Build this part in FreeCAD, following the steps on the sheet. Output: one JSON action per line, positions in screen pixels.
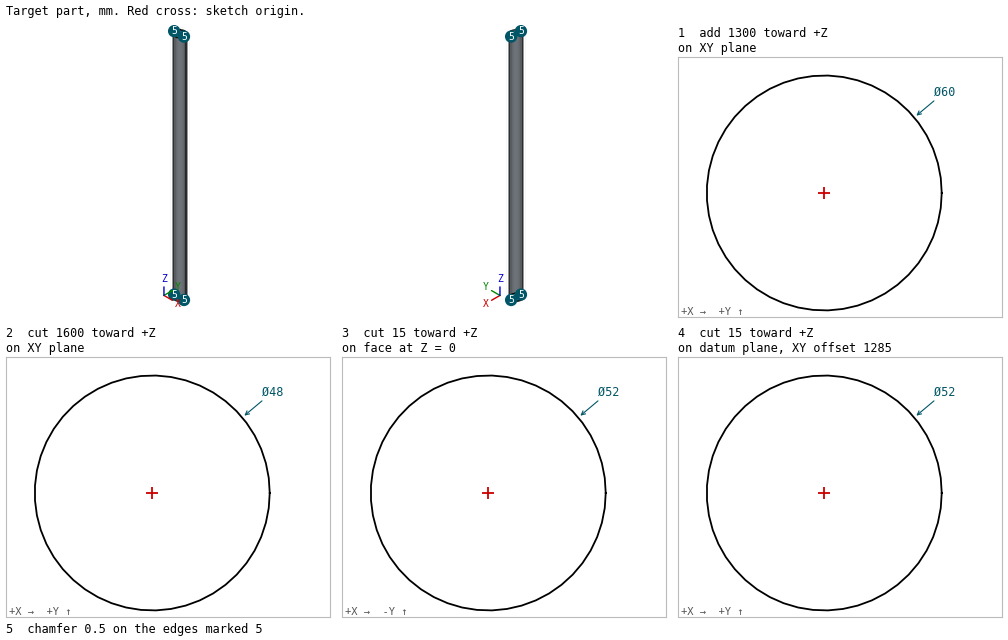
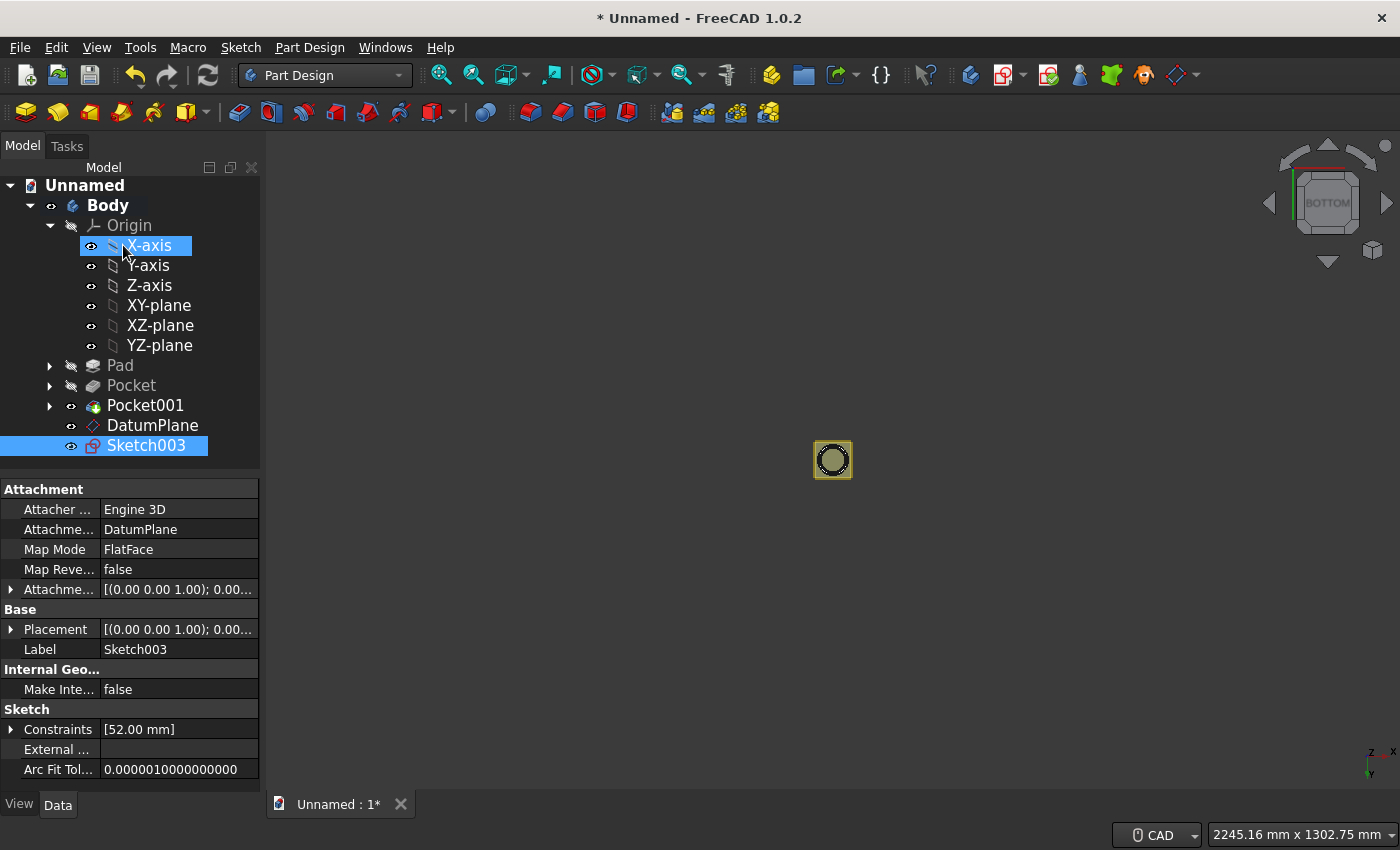
{"action": "left_click", "coordinate": [240, 112]}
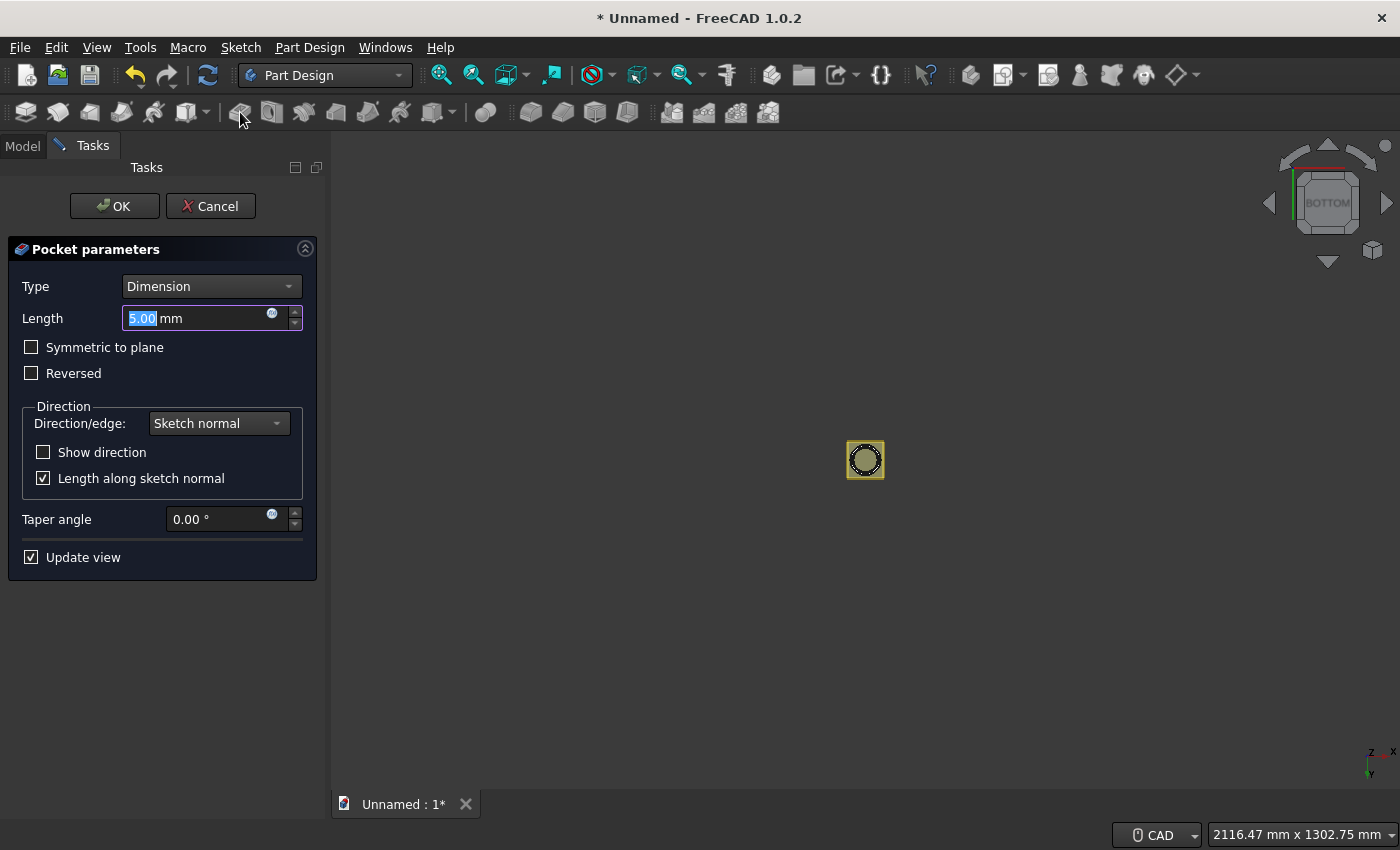
{"action": "type", "text": "15"}
{"action": "key", "text": "Tab"}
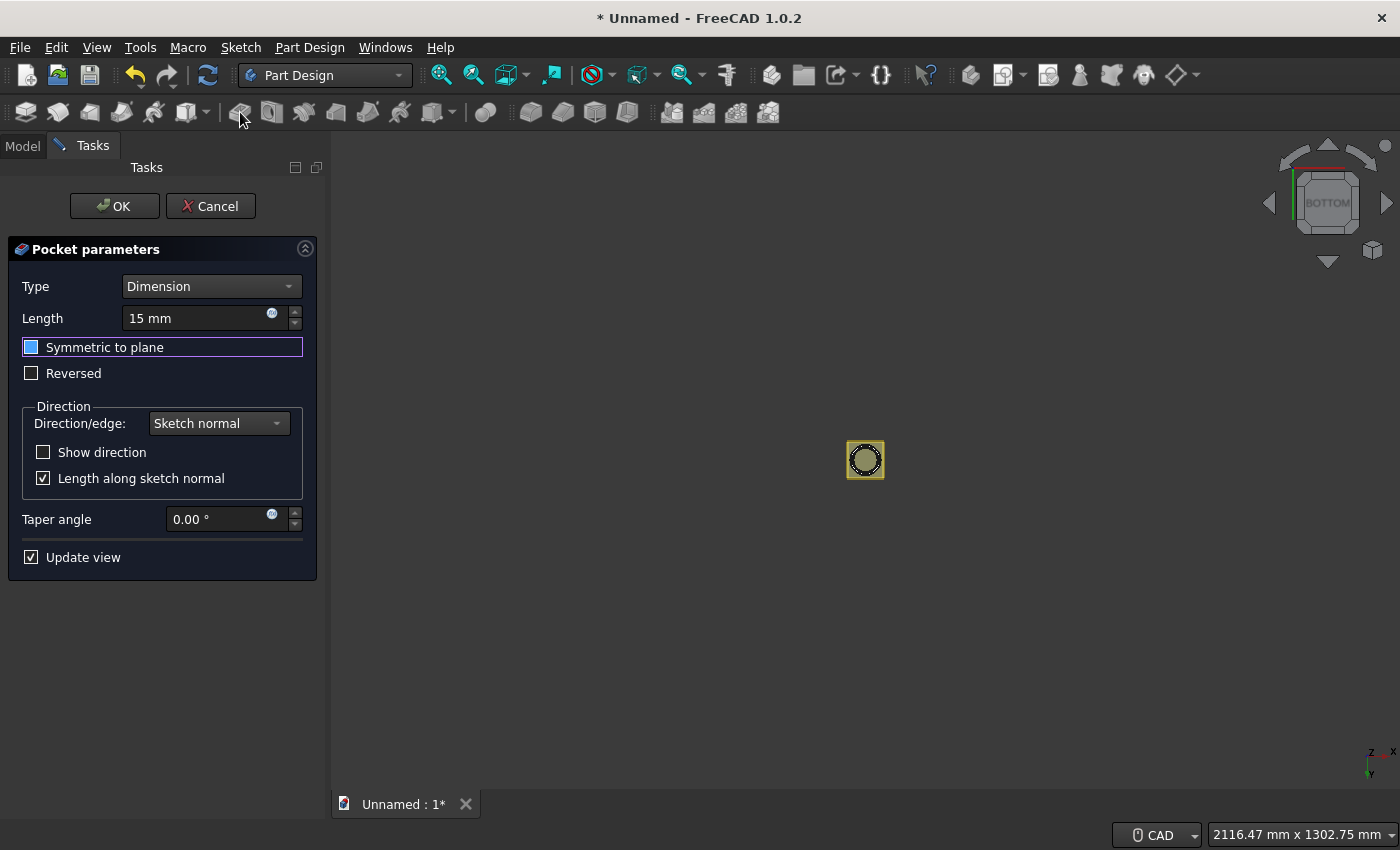
{"action": "left_click", "coordinate": [30, 373]}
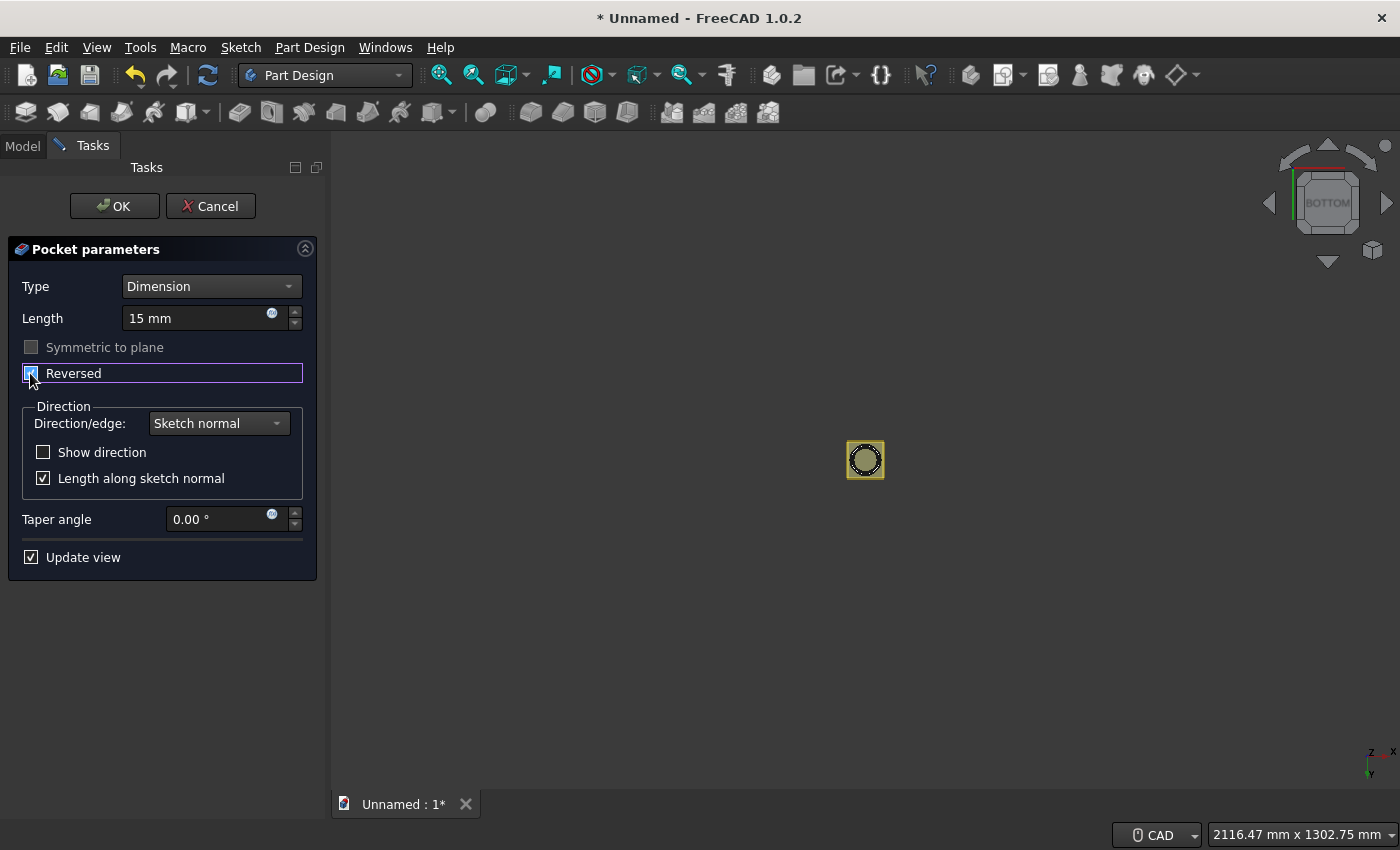
{"action": "left_click", "coordinate": [115, 206]}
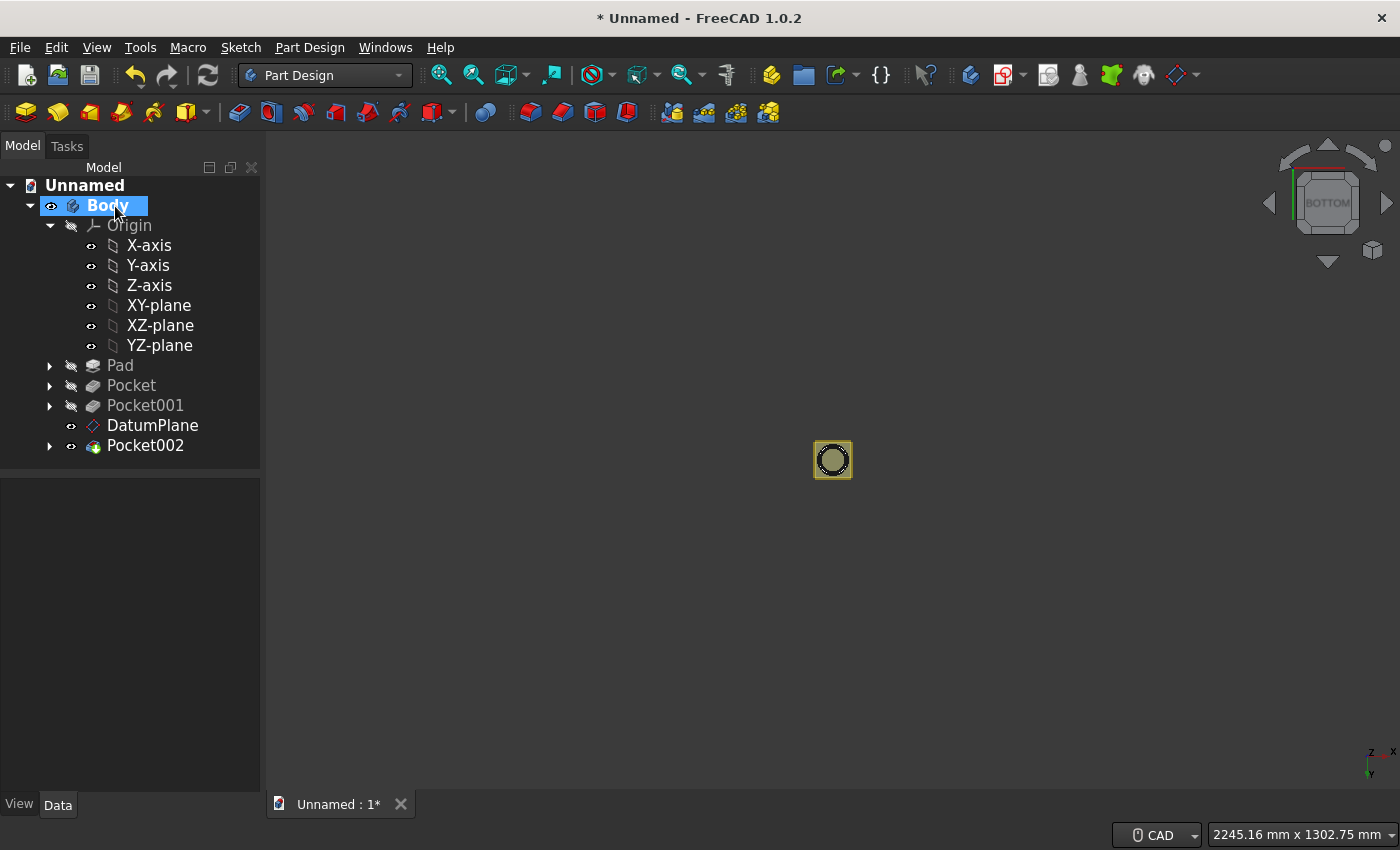
{"action": "left_click", "coordinate": [116, 426]}
{"action": "key", "text": "space"}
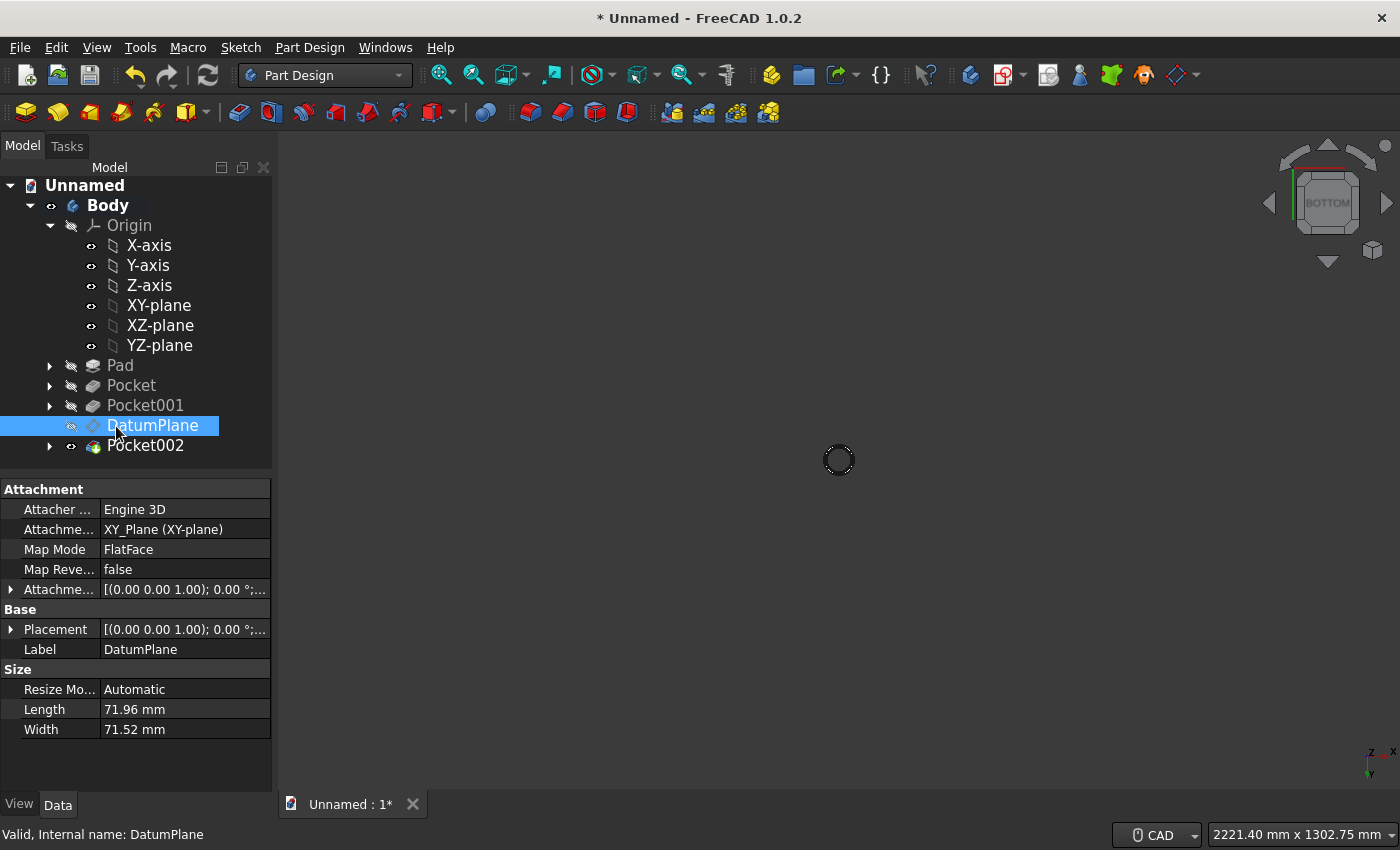
{"action": "left_click", "coordinate": [442, 76]}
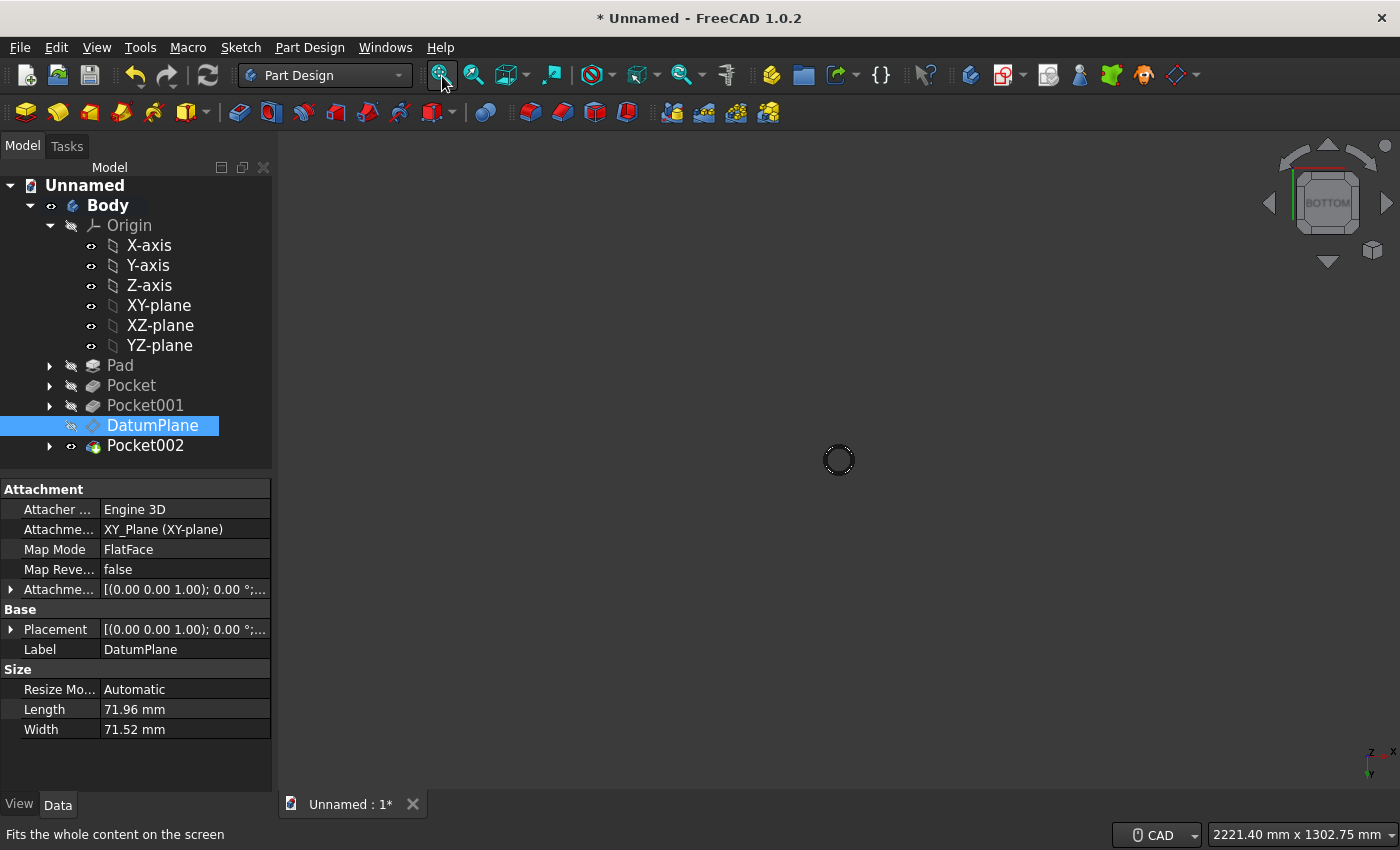
{"action": "left_click", "coordinate": [828, 451]}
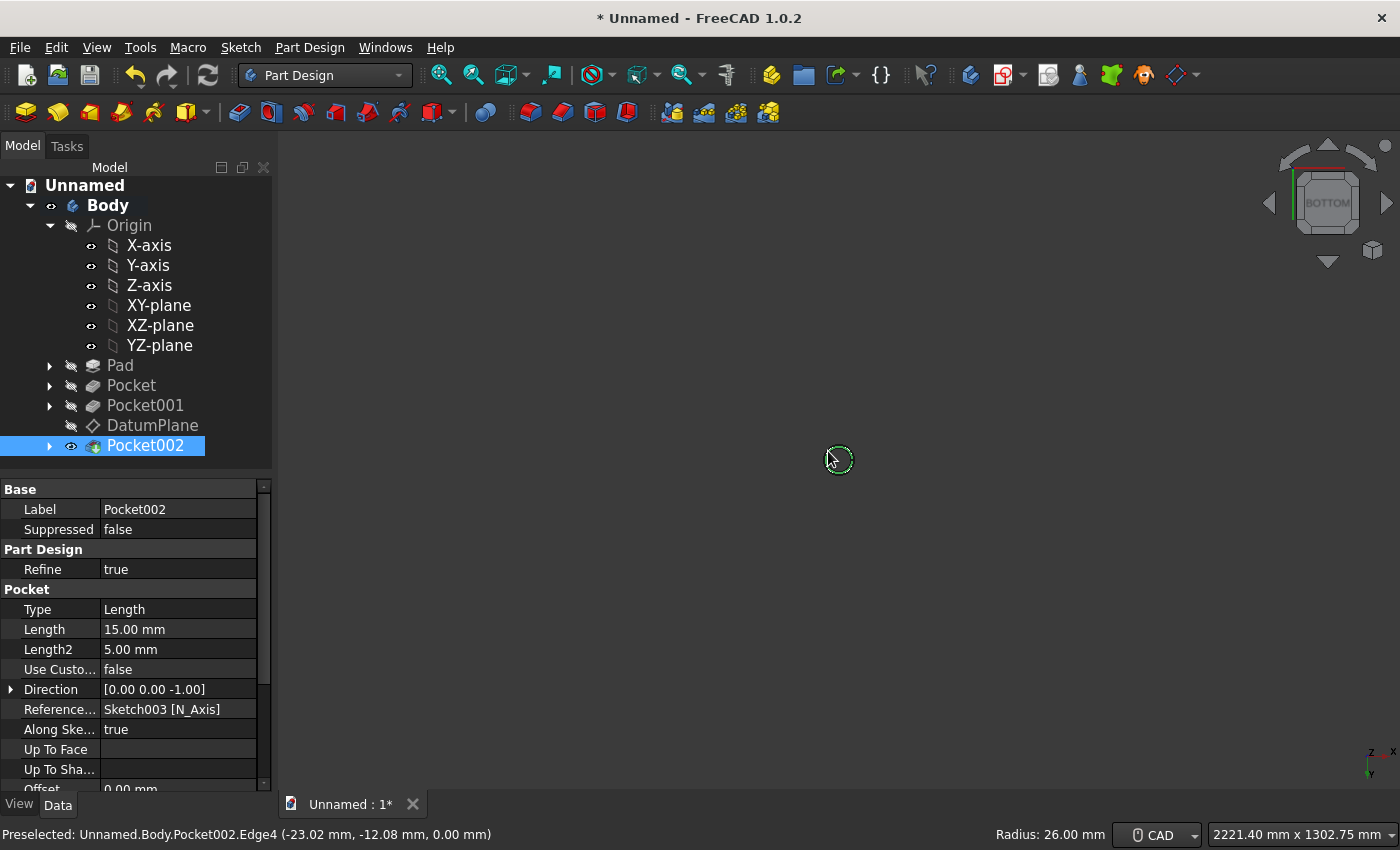
{"action": "left_click", "coordinate": [824, 459], "text": "ctrl"}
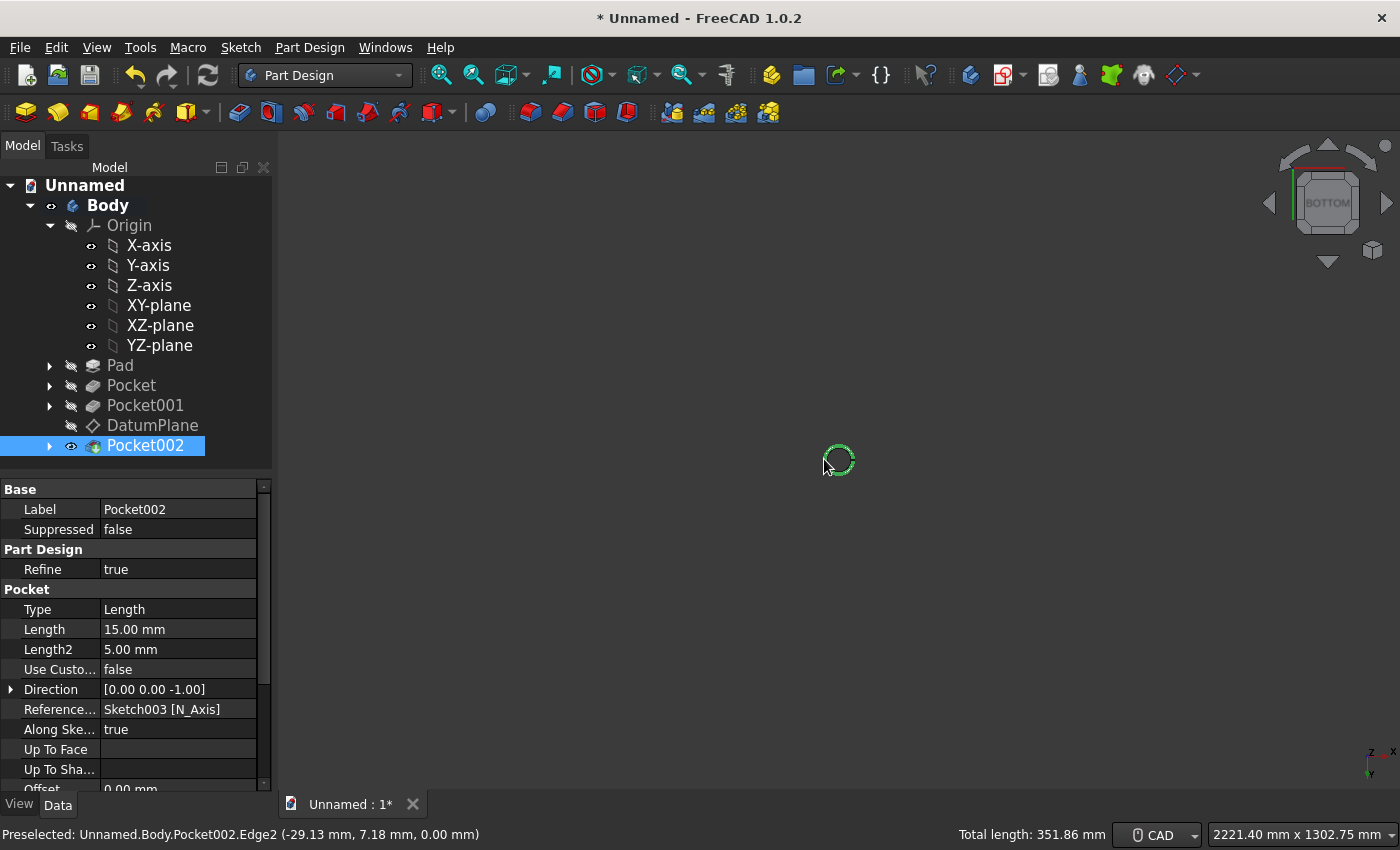
{"action": "key", "text": "0"}